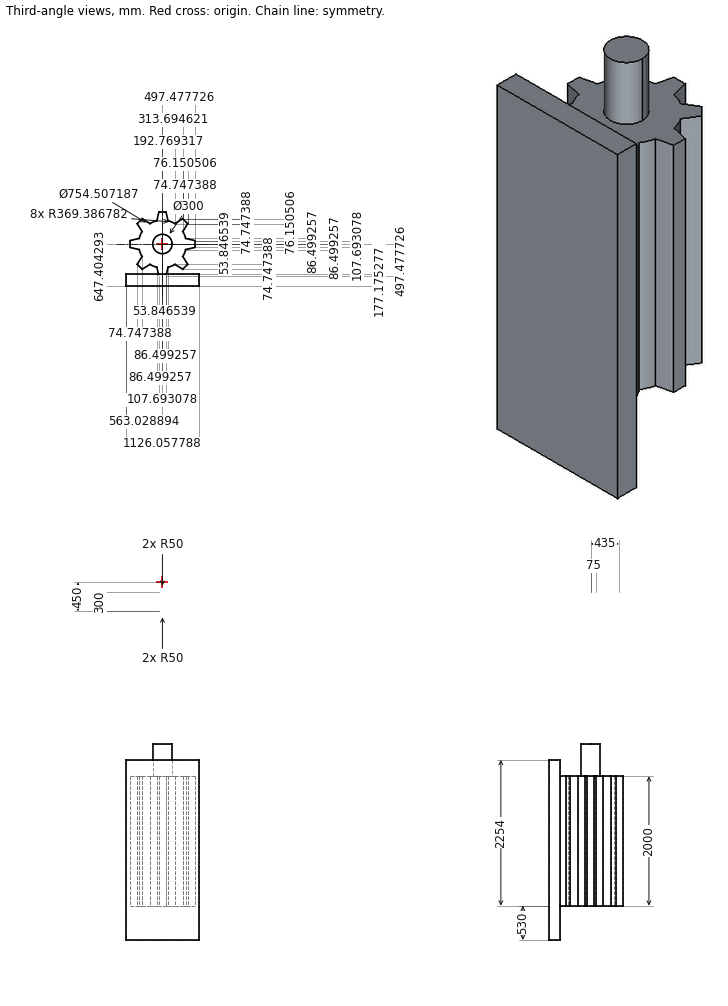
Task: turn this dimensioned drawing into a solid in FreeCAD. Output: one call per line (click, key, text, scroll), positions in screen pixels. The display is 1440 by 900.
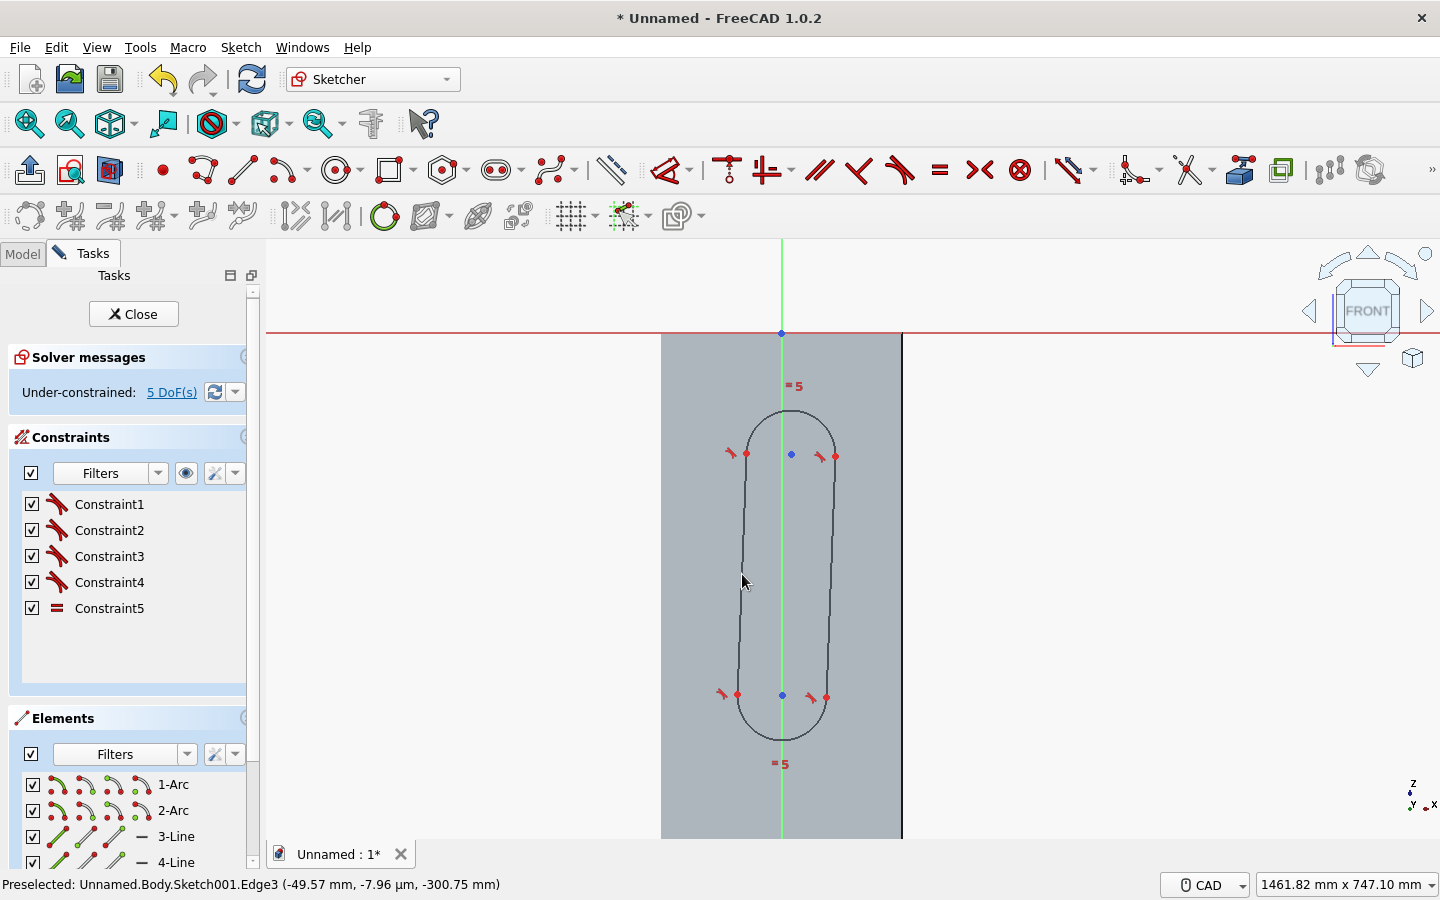
click(740, 622)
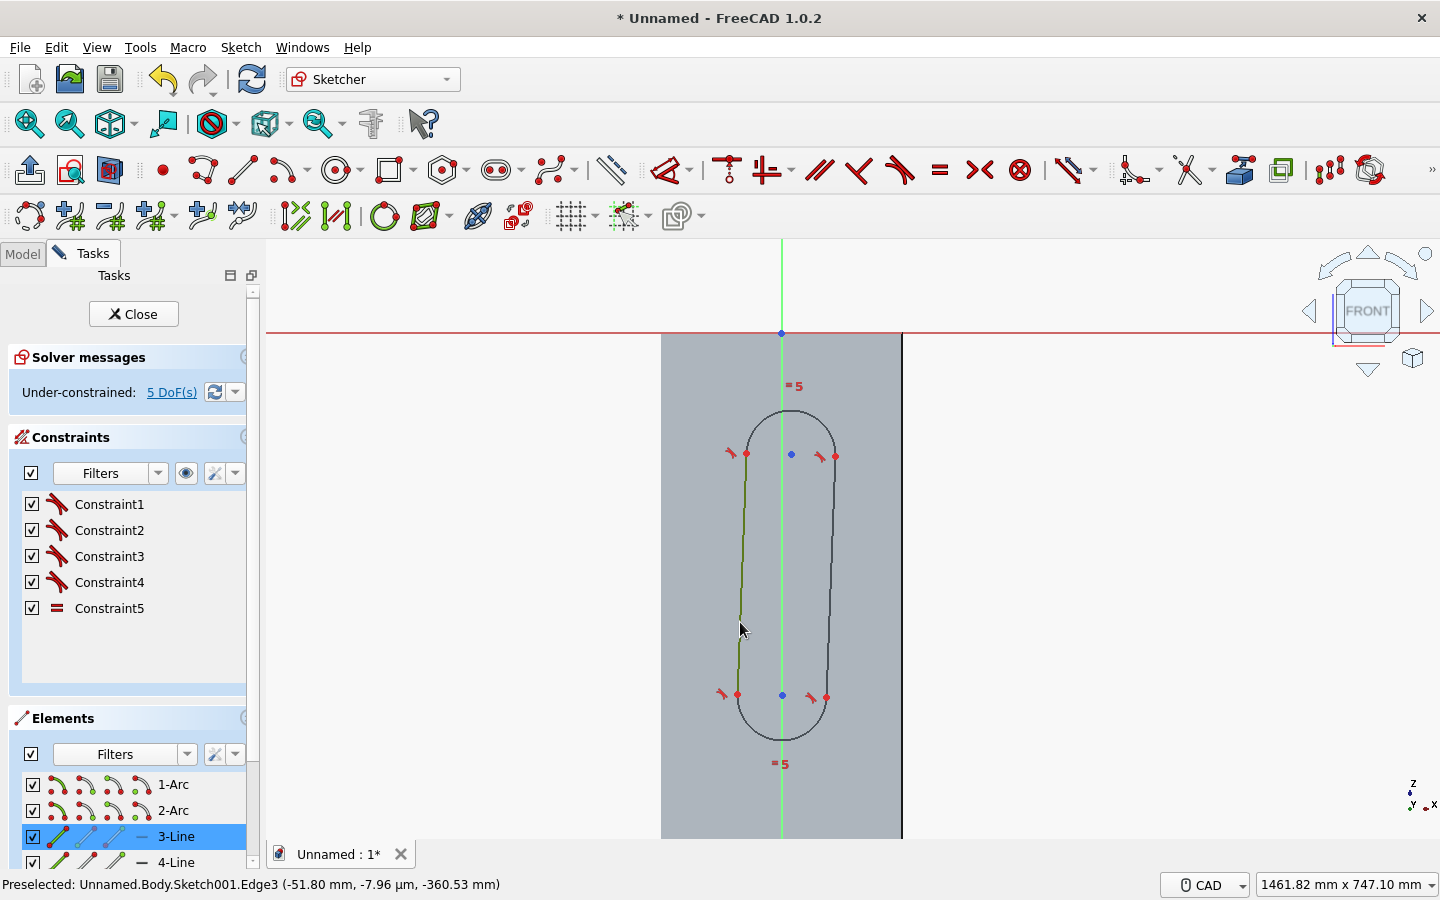
key(v)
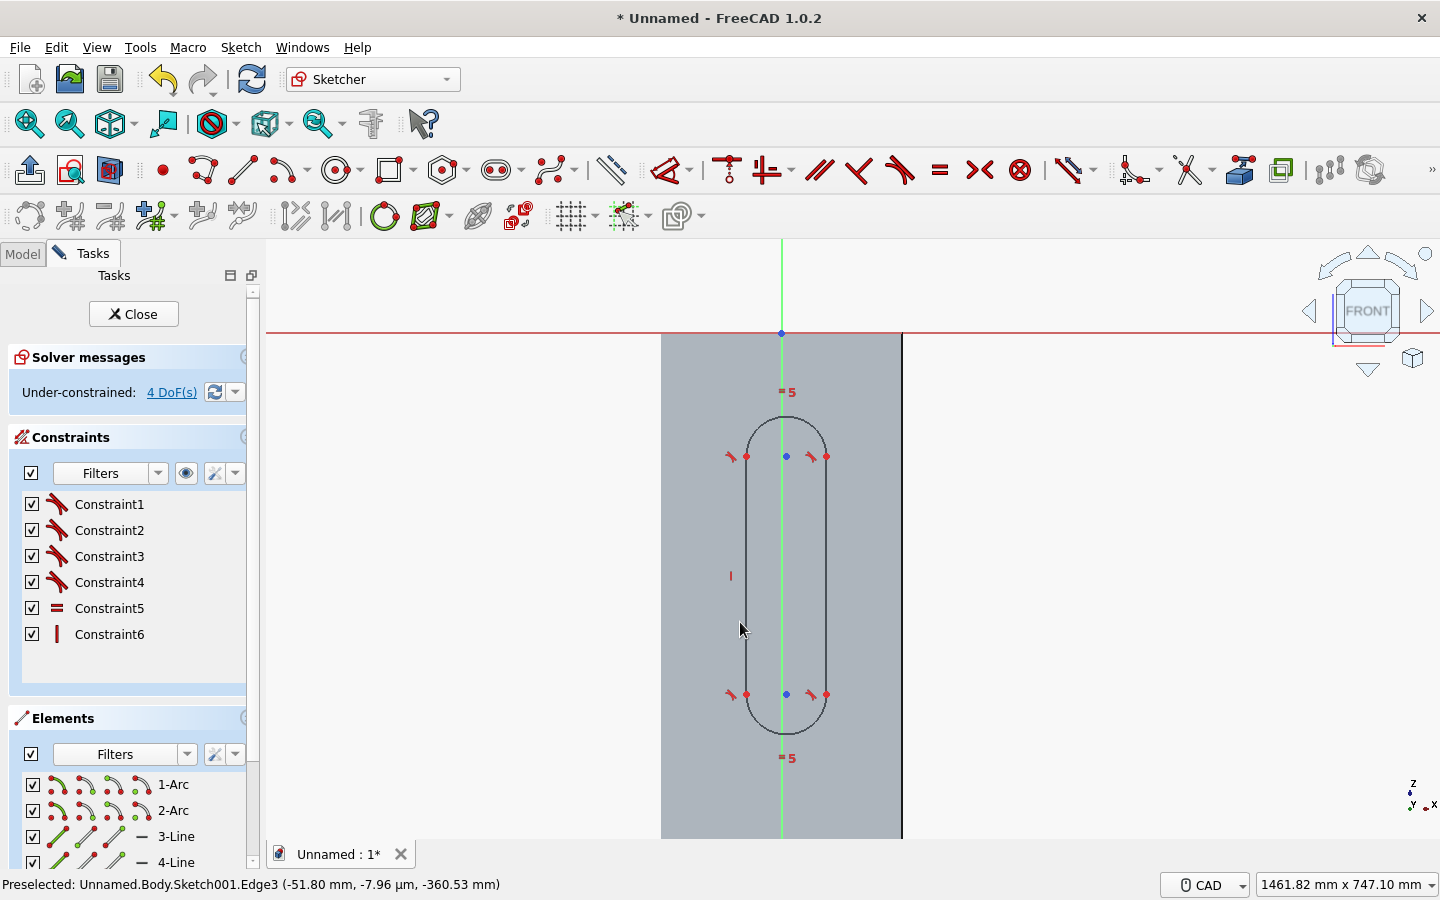
click(786, 694)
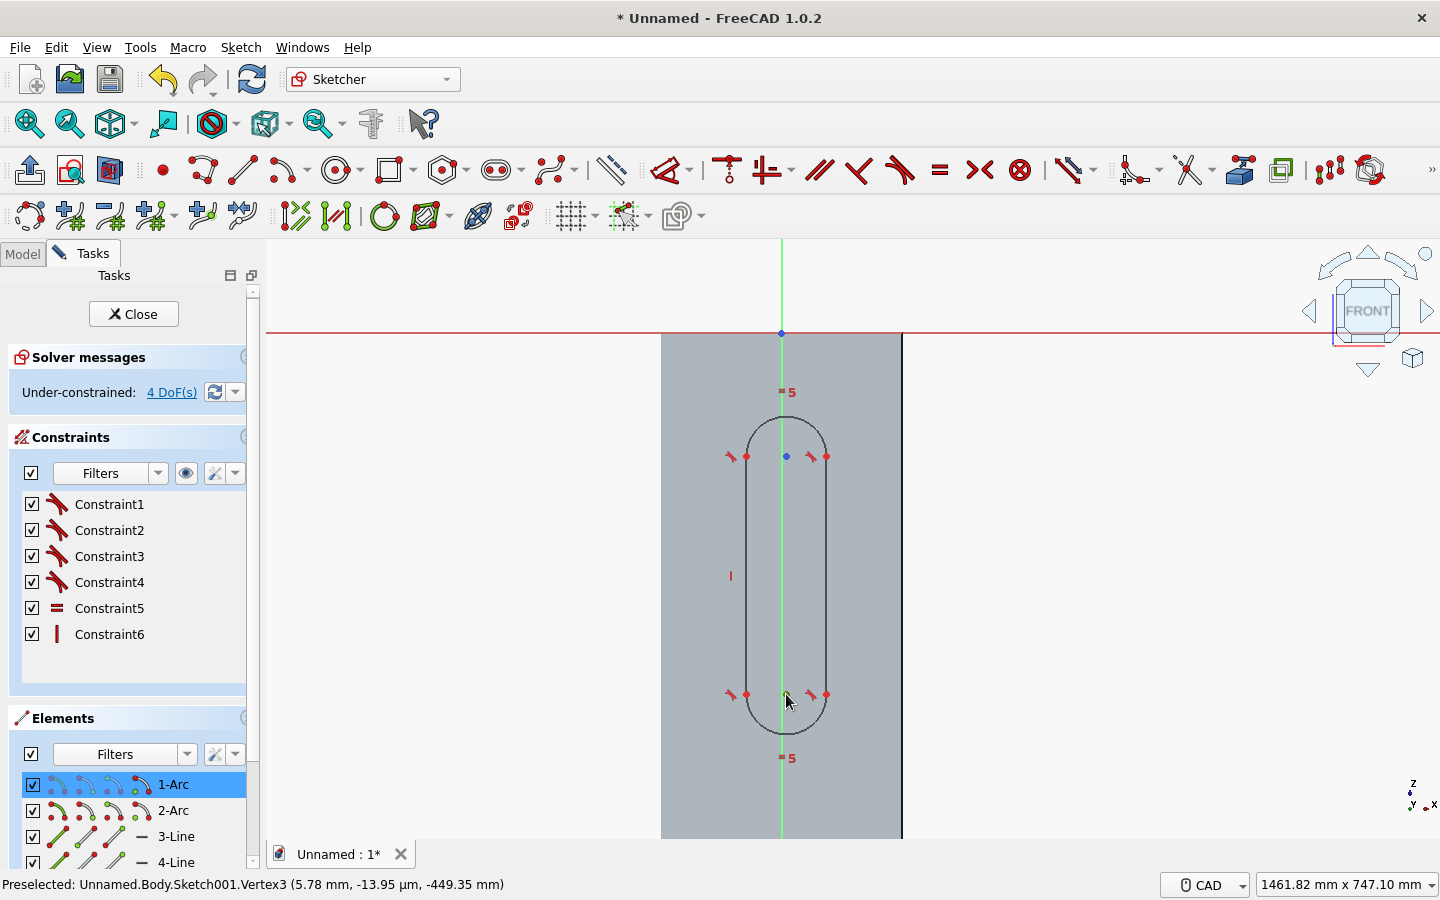
click(782, 772)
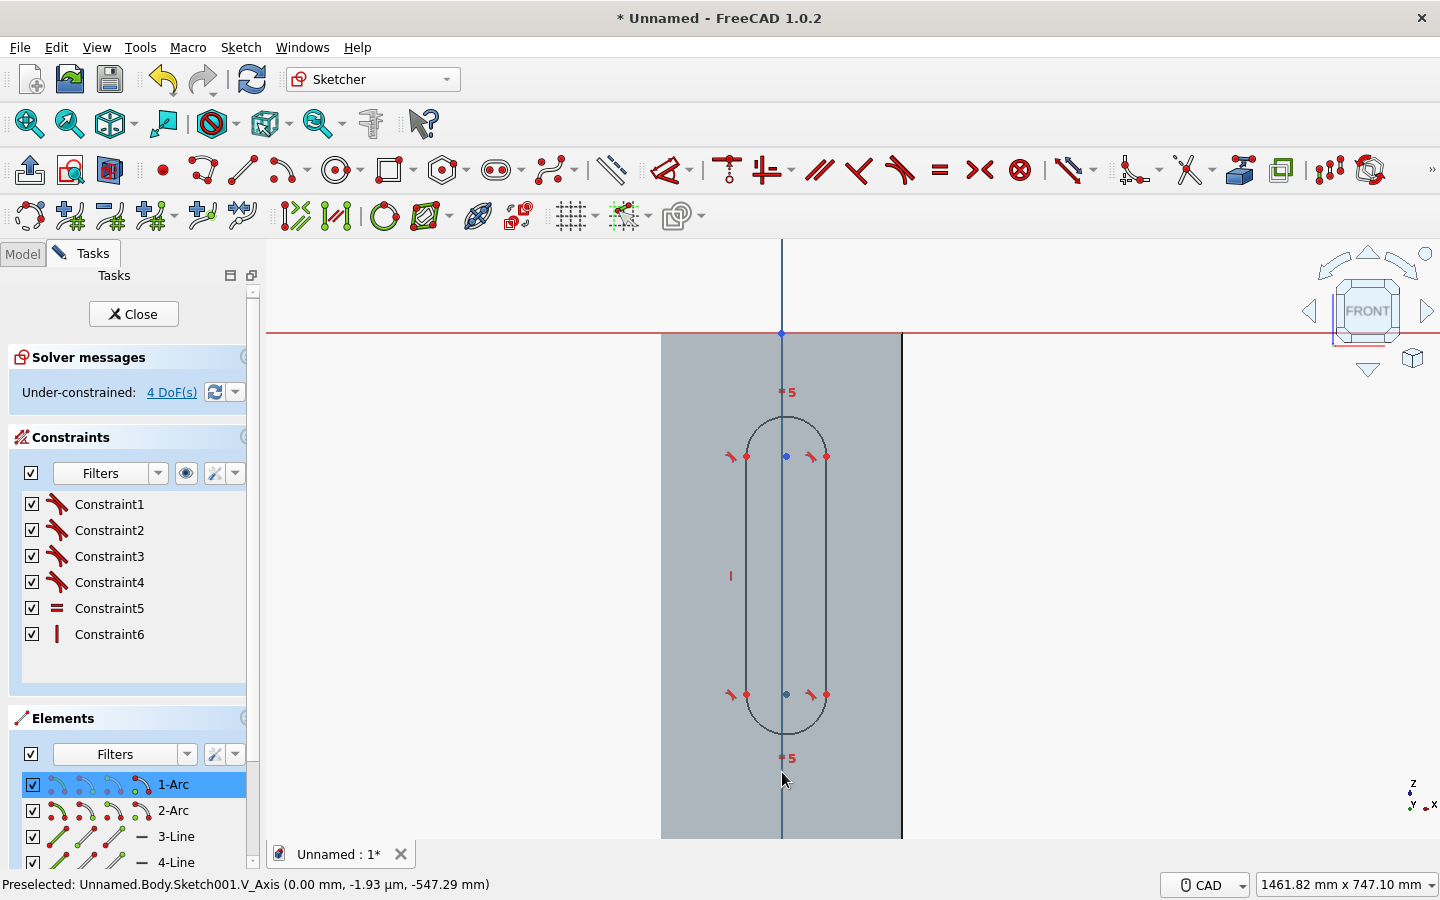
click(728, 170)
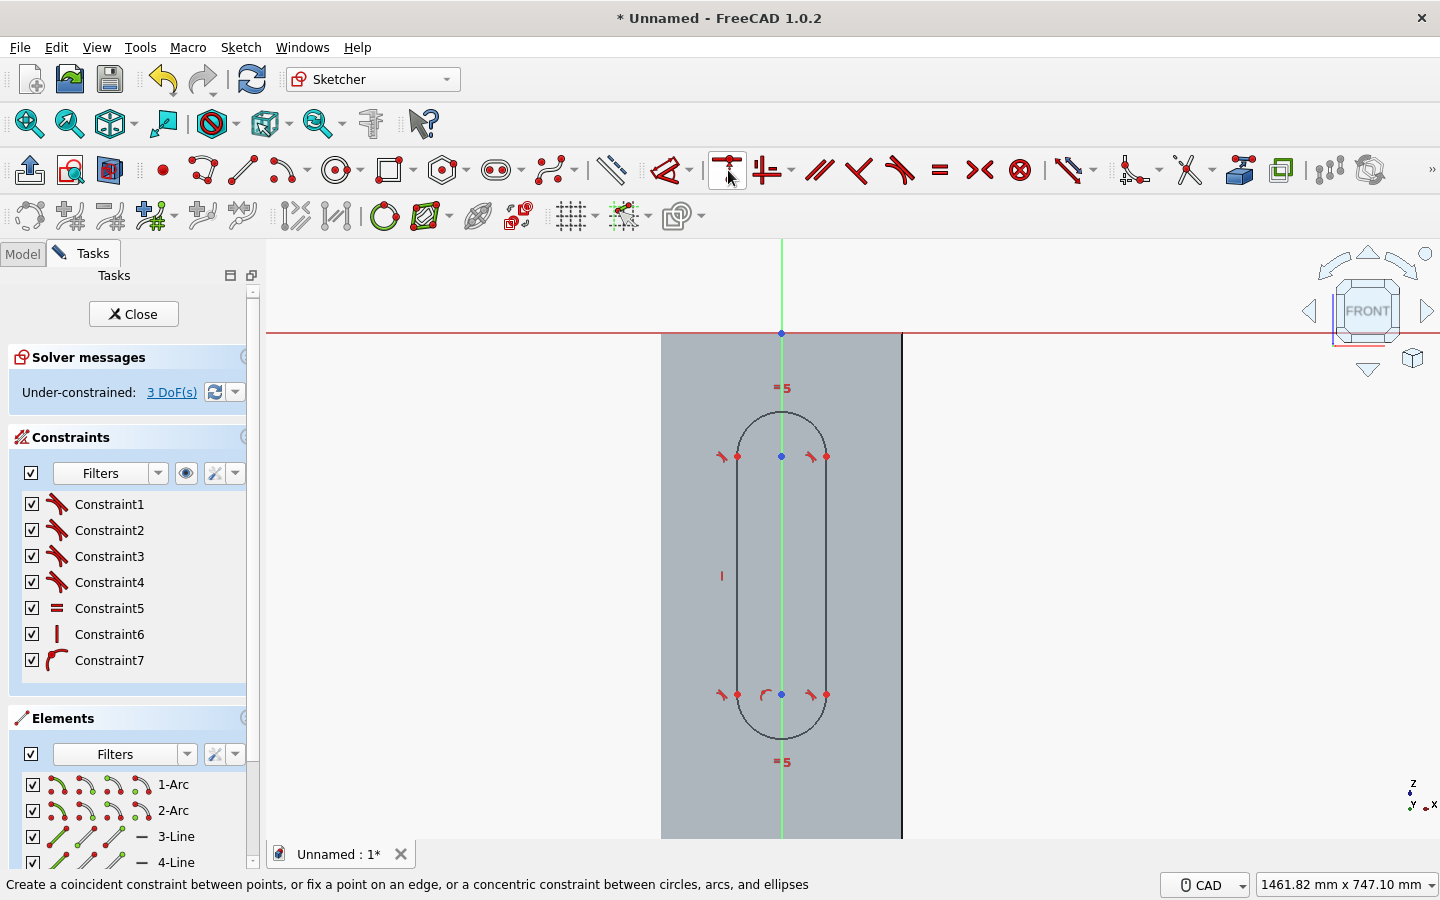
click(666, 170)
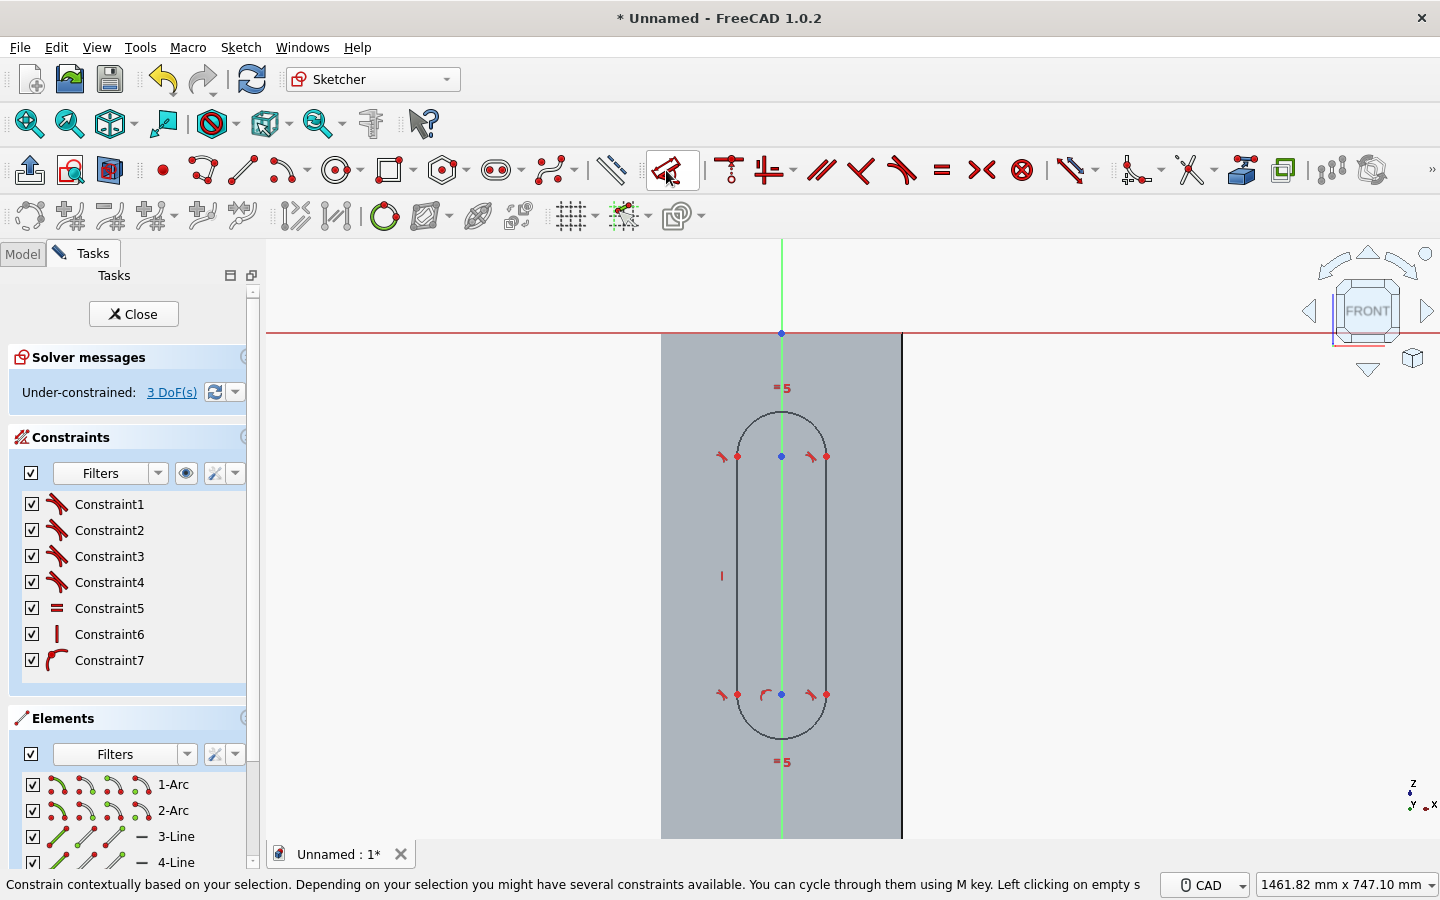
click(756, 730)
click(737, 756)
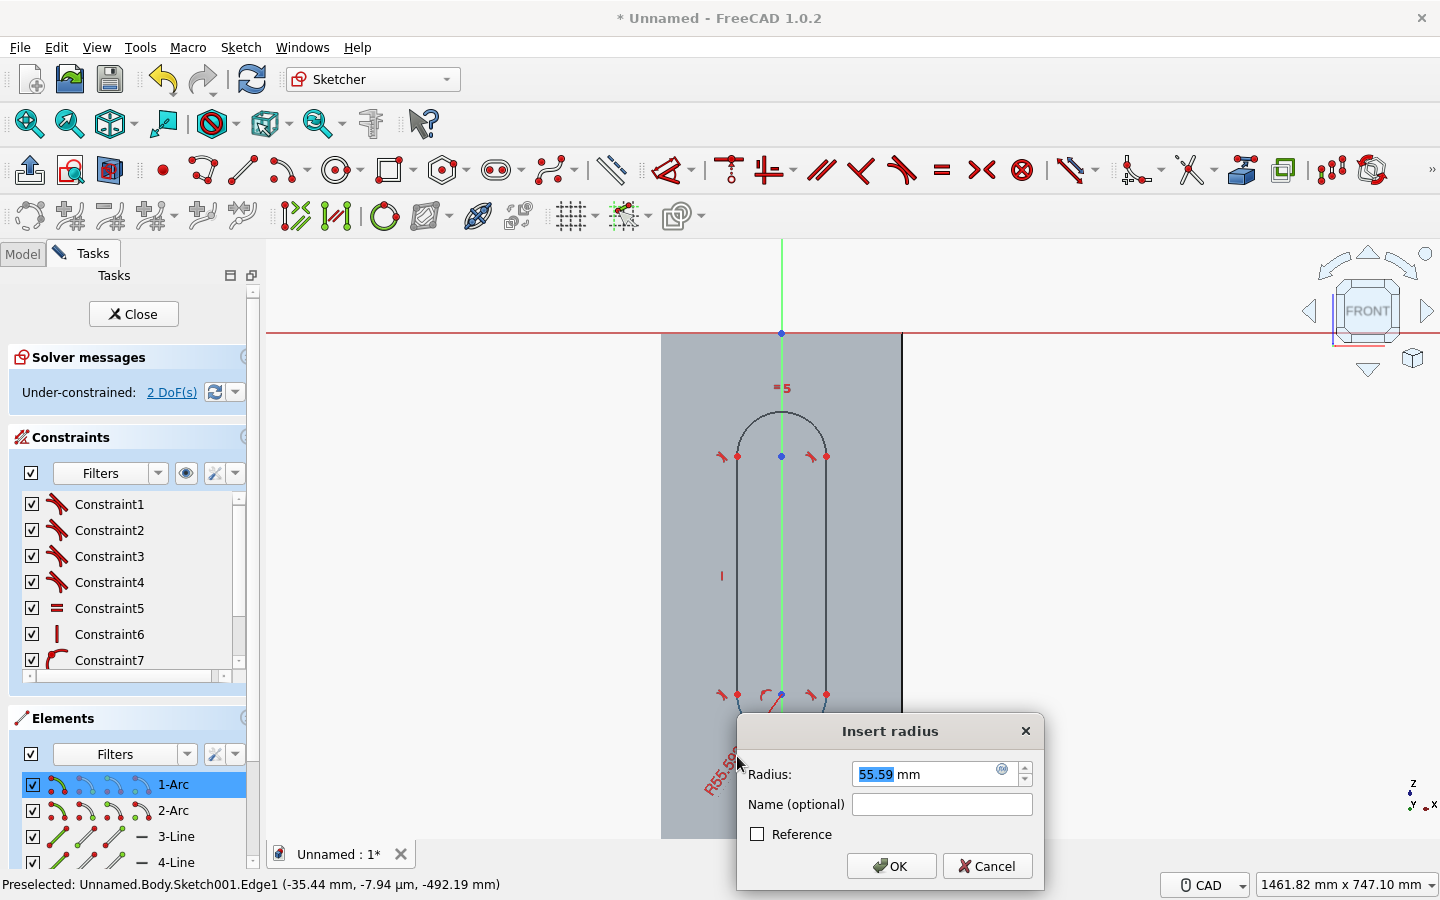
text(50)
key(Return)